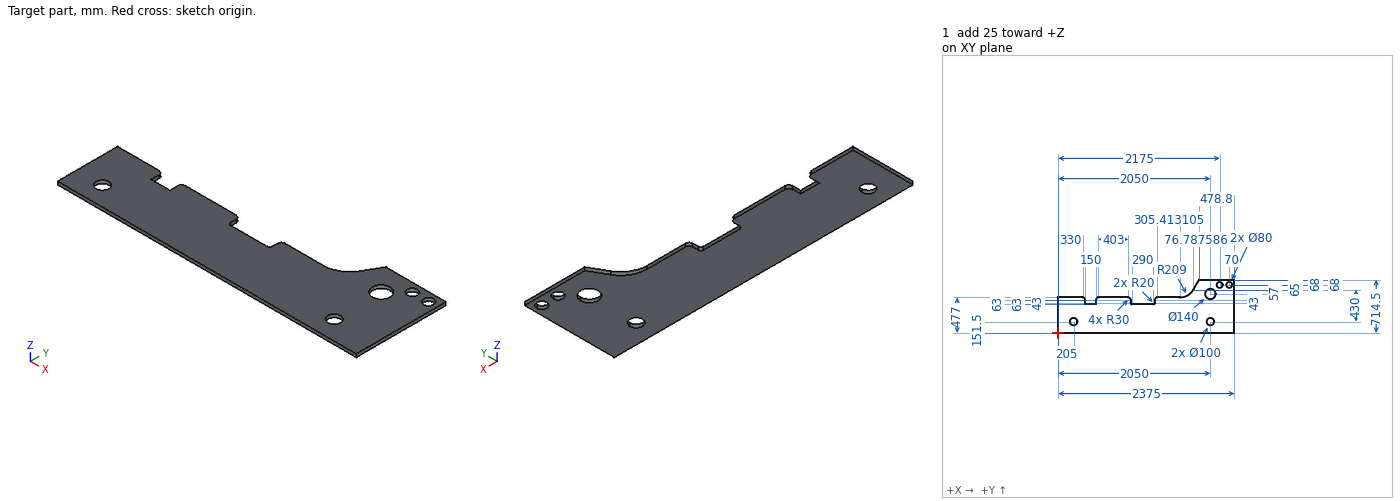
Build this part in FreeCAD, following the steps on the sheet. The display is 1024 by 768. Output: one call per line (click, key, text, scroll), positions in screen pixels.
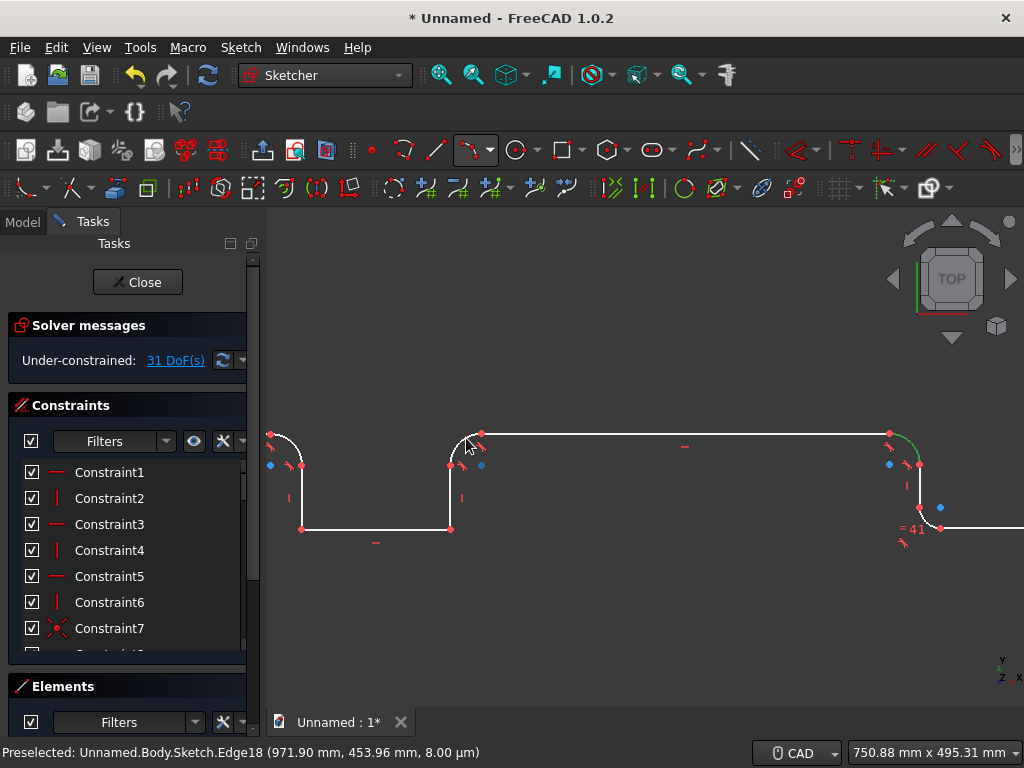
click(468, 437)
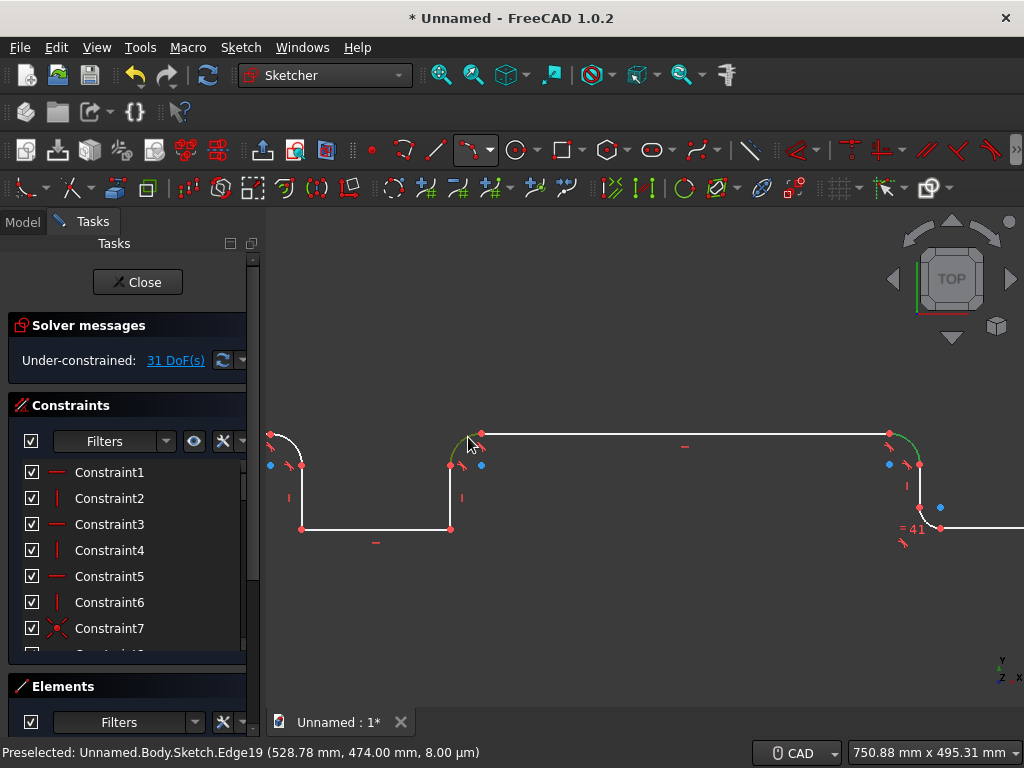
click(299, 451)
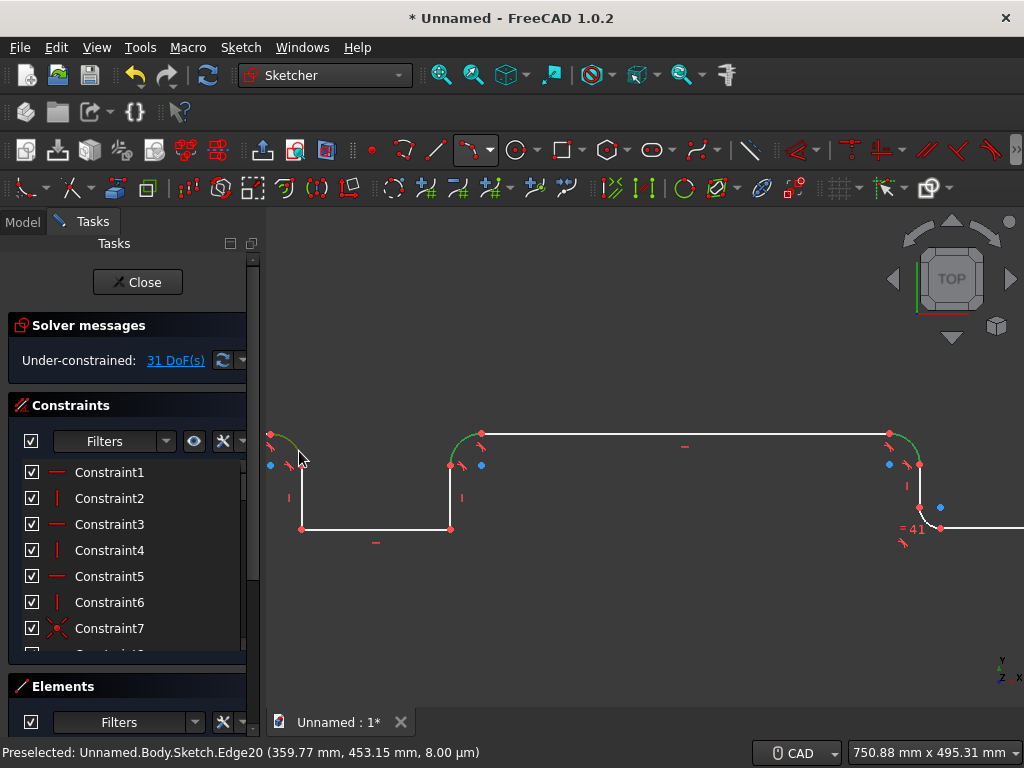
key(e)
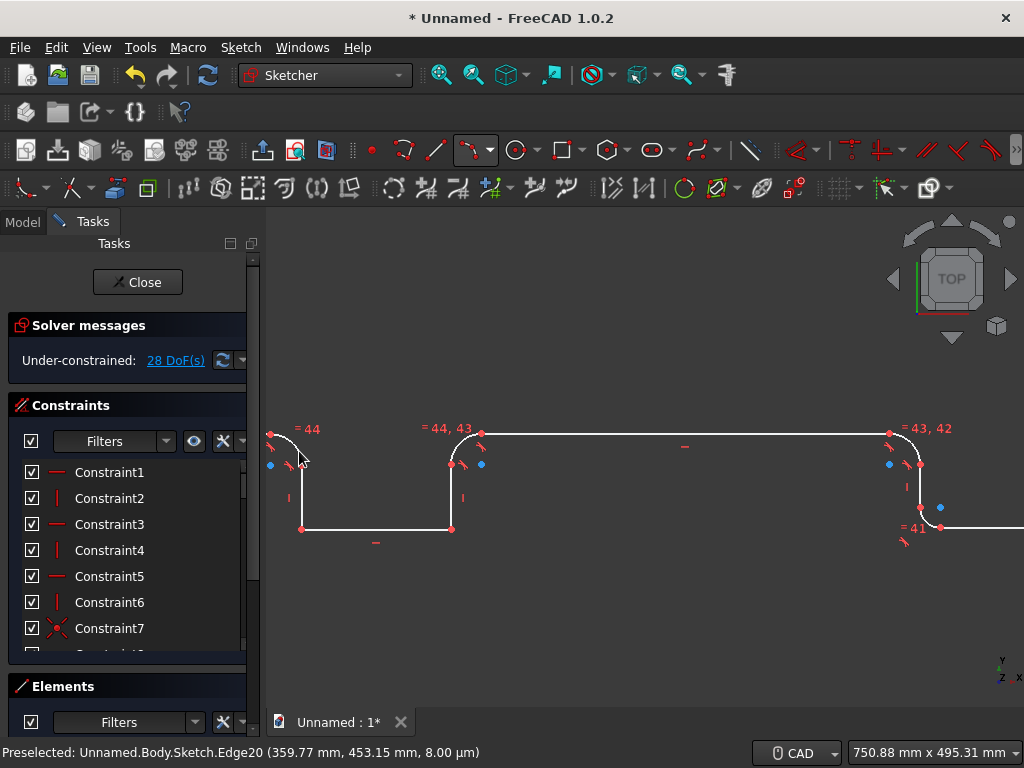
click(796, 150)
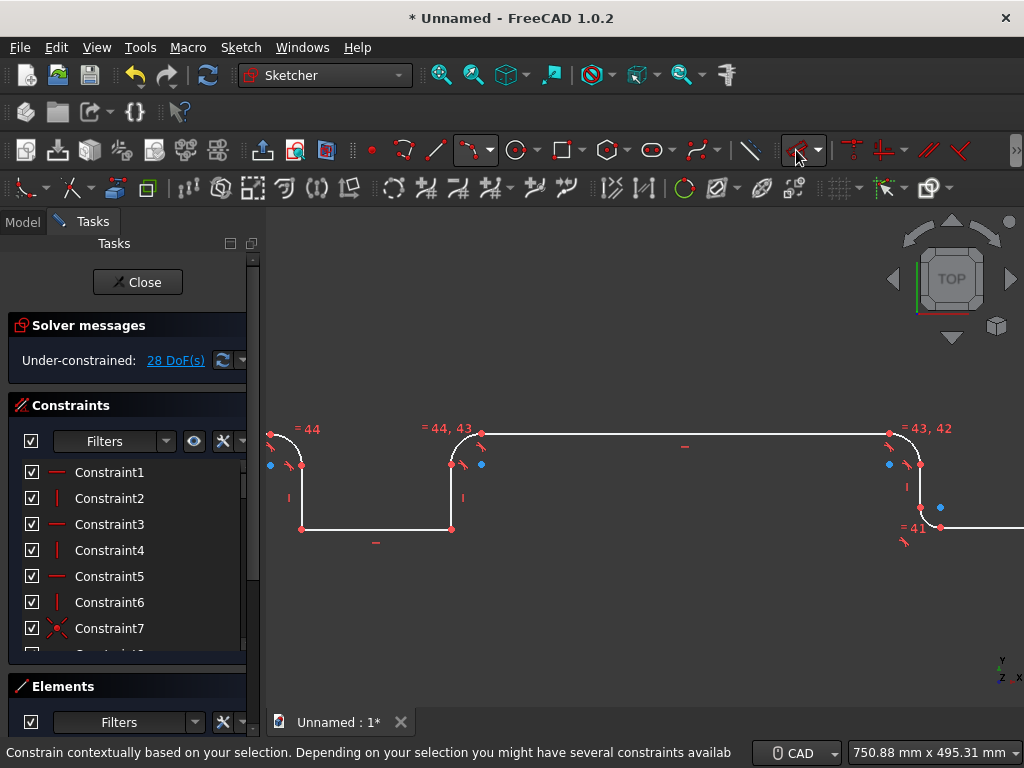
scroll(466, 438, down, 9)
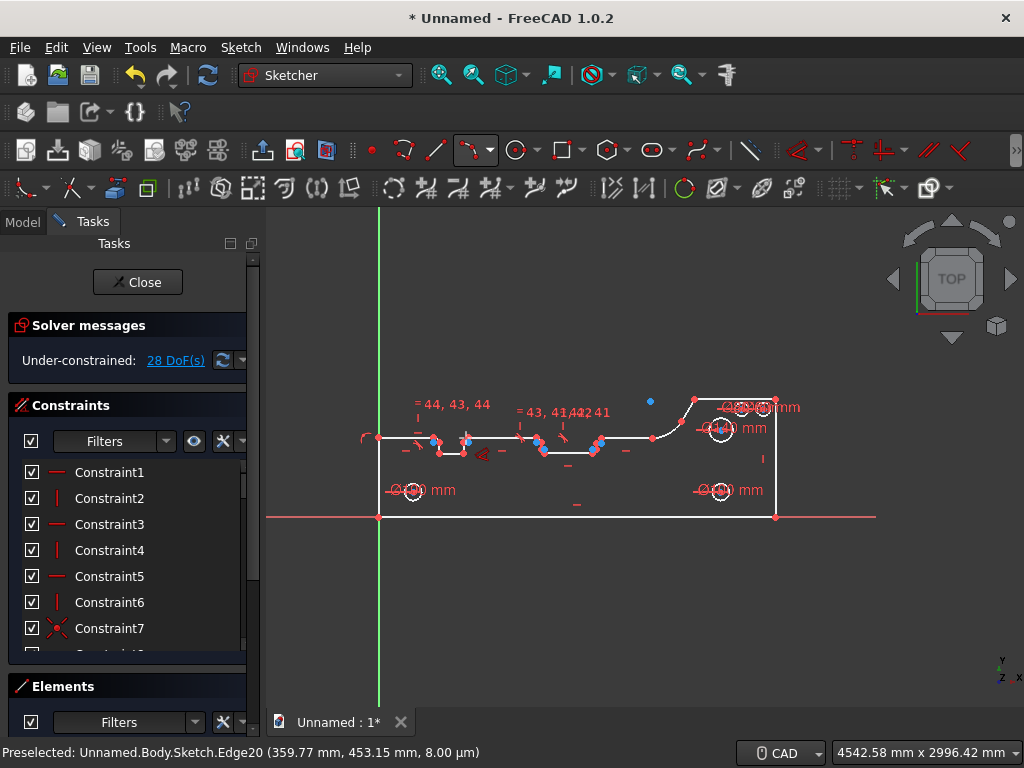
scroll(599, 439, up, 11)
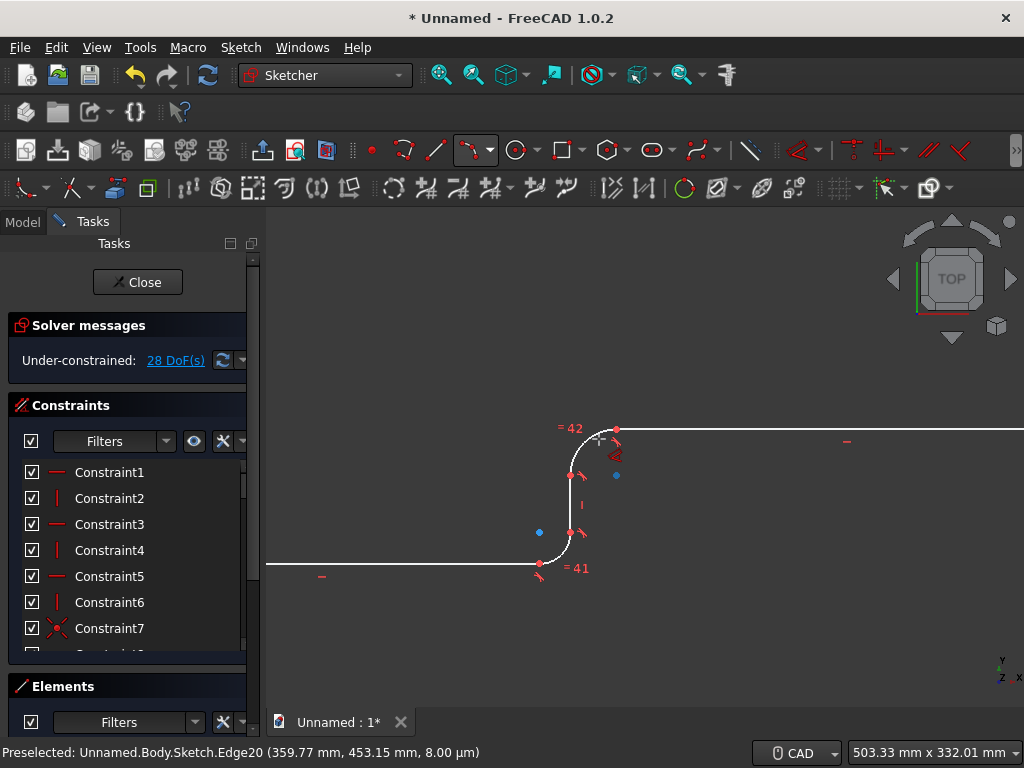
click(596, 435)
click(582, 406)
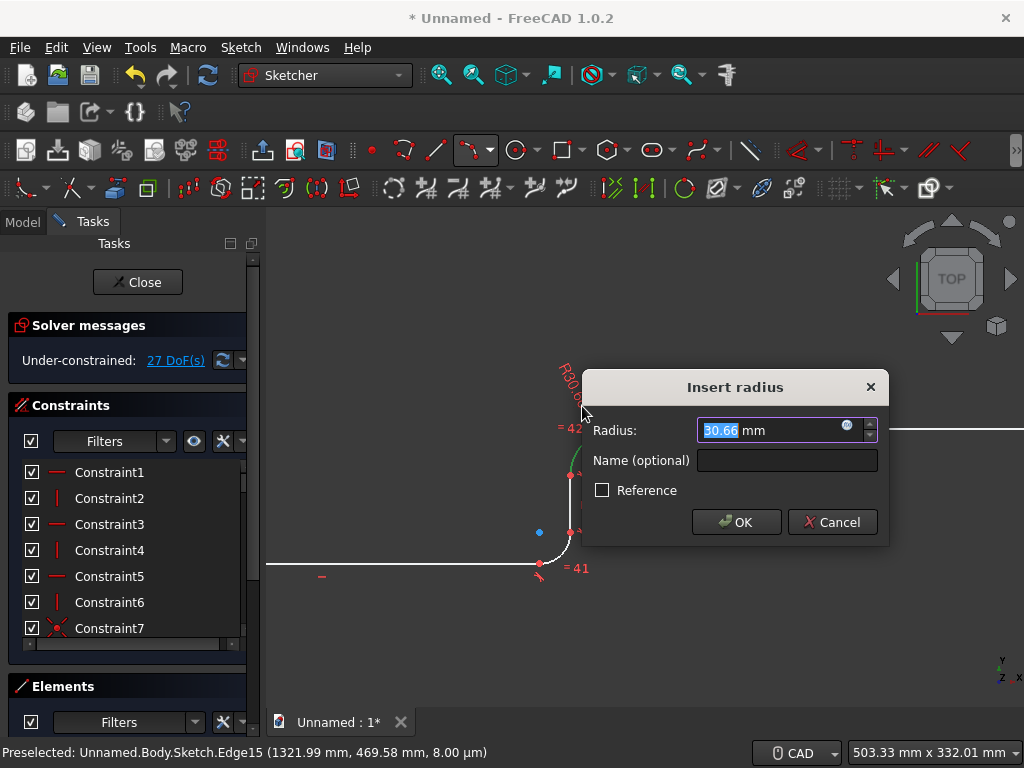
text(30)
key(Return)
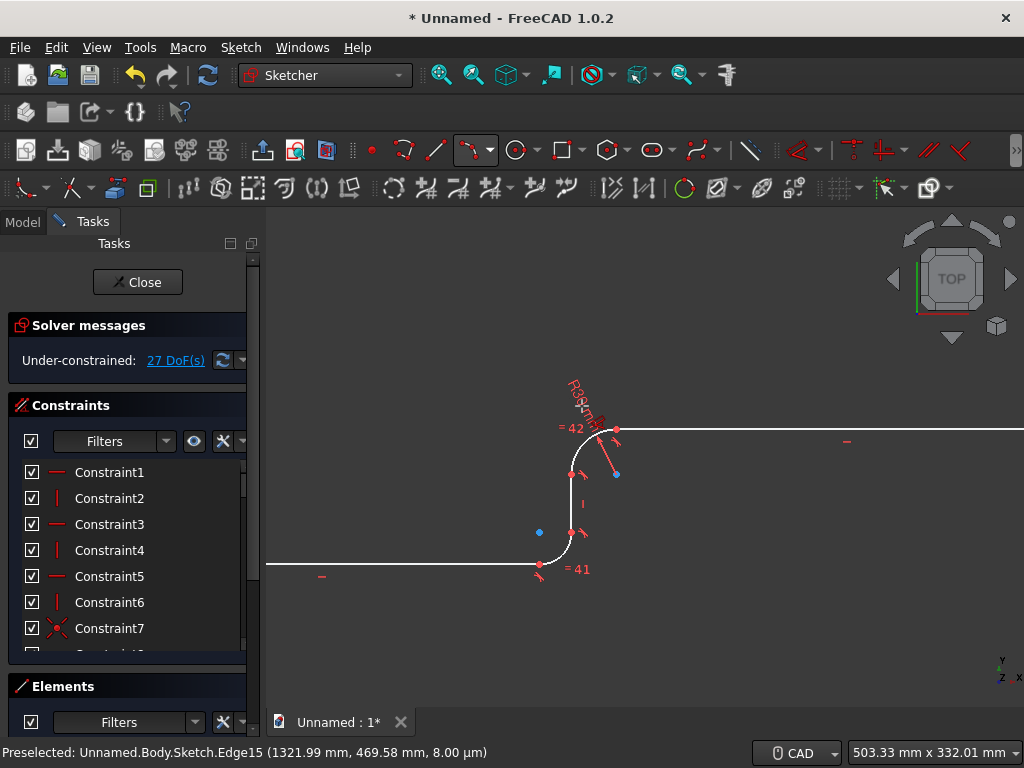
scroll(554, 561, up, 2)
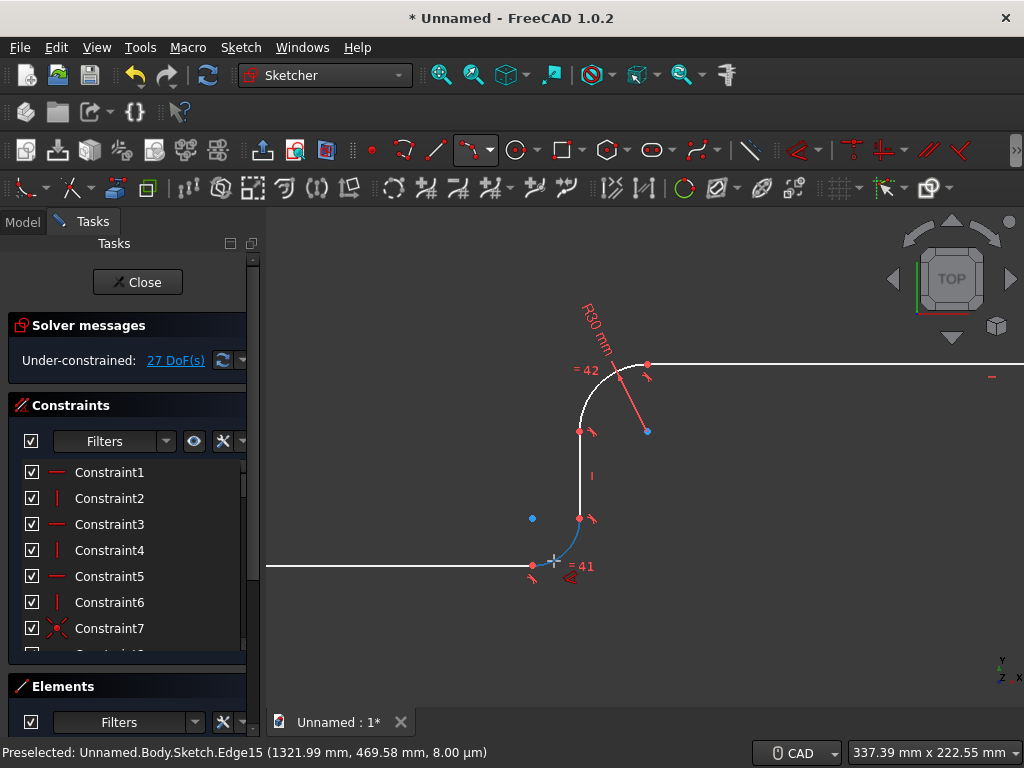
click(554, 561)
click(568, 590)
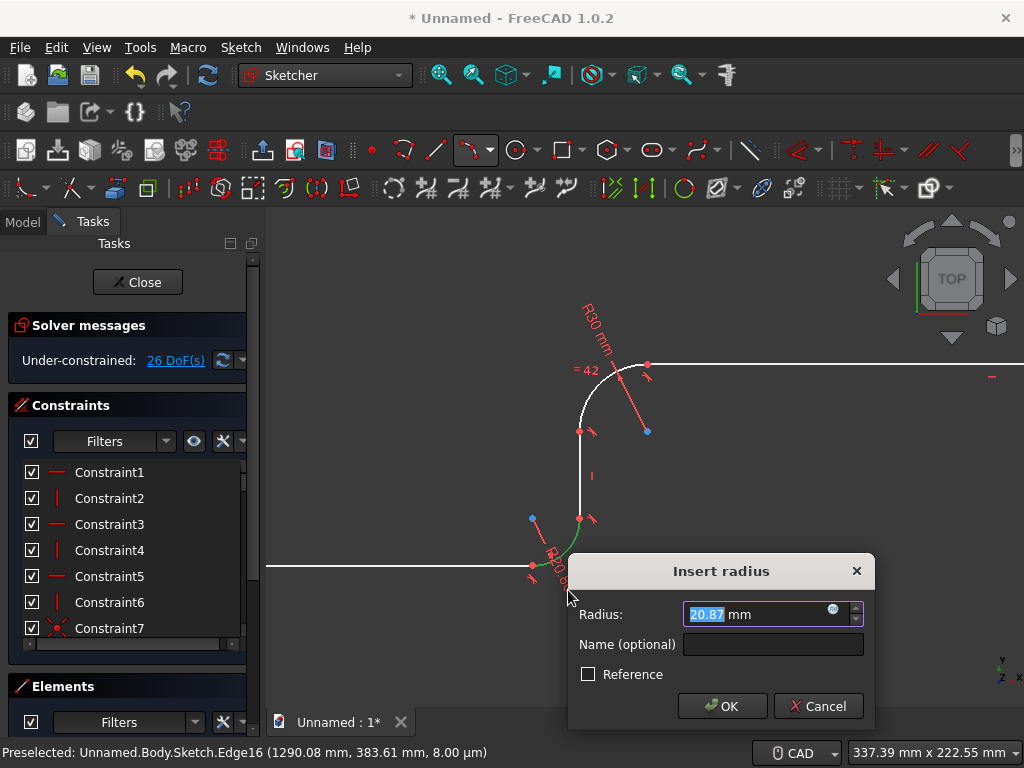
text(20)
key(Return)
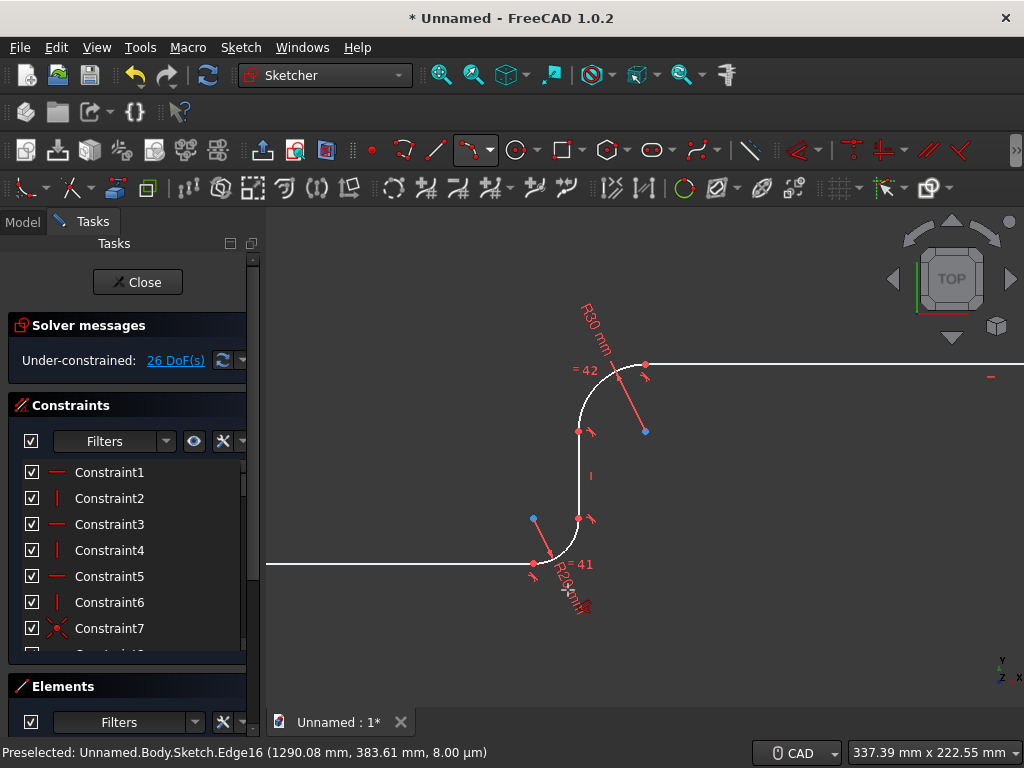
scroll(597, 444, down, 13)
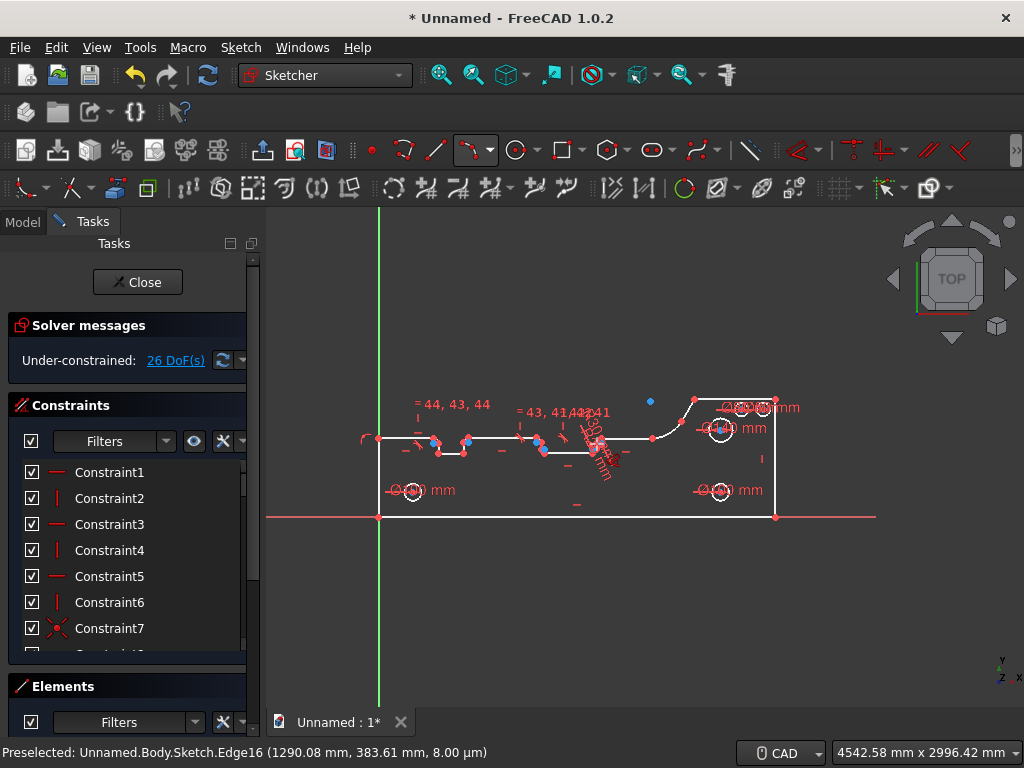
scroll(663, 436, up, 2)